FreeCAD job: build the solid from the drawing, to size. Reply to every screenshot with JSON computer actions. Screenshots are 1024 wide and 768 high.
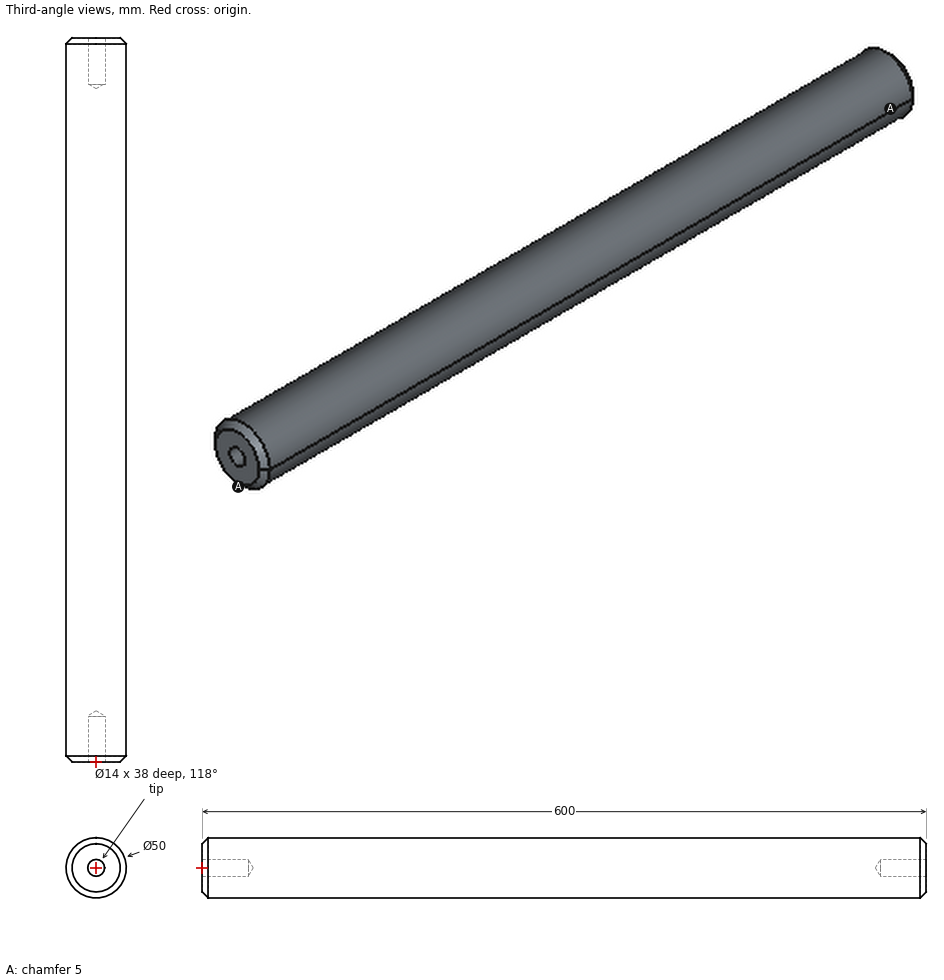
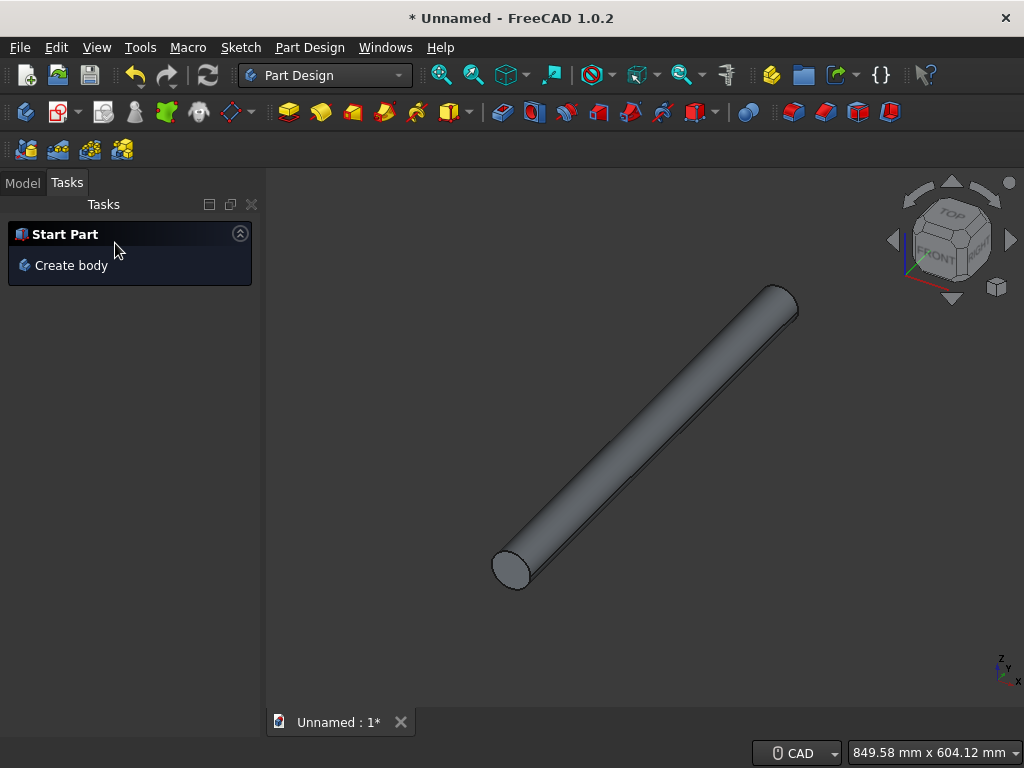
{"action": "left_click", "coordinate": [496, 554]}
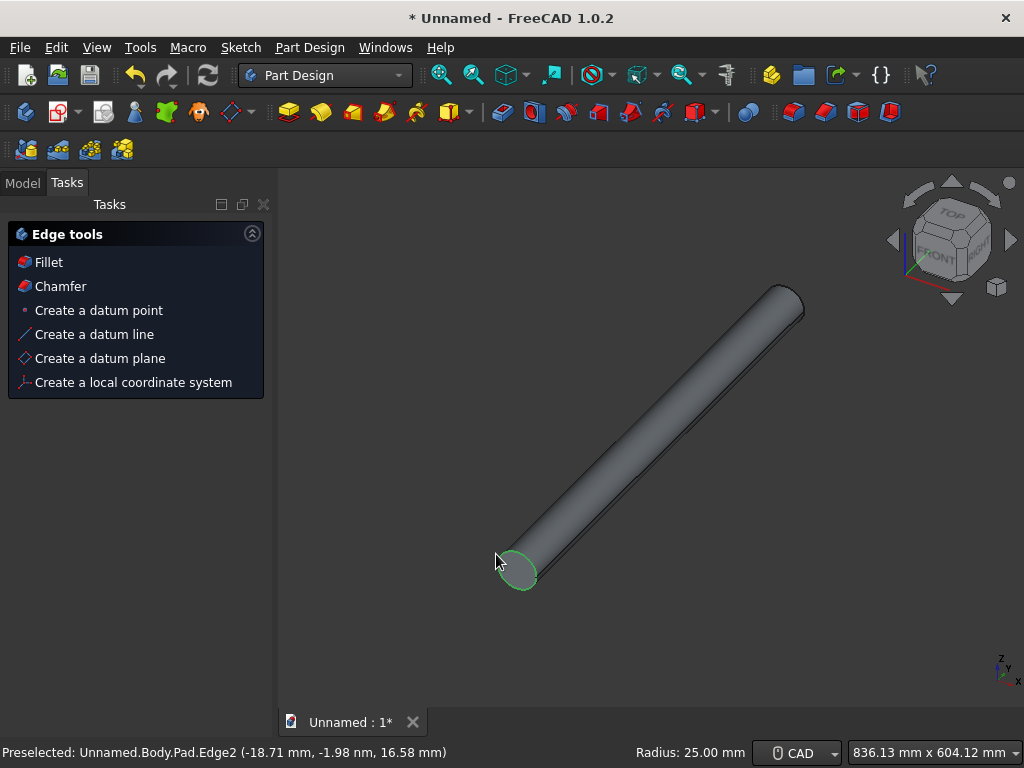
{"action": "left_click", "coordinate": [779, 284], "text": "ctrl"}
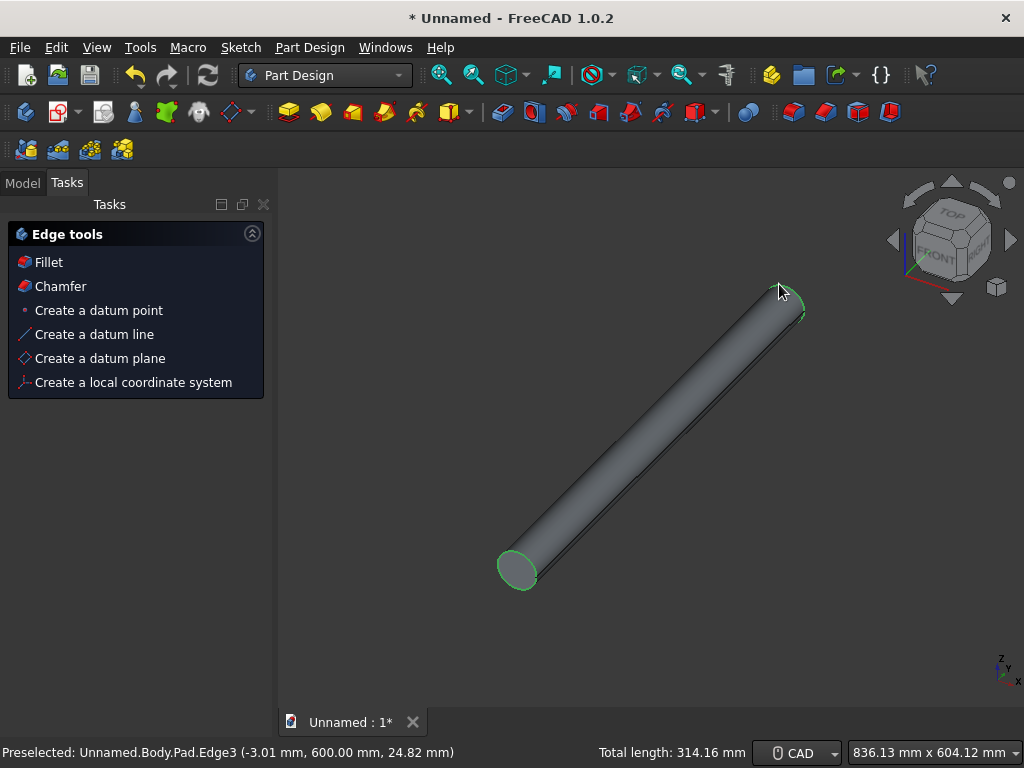
{"action": "left_click", "coordinate": [826, 112]}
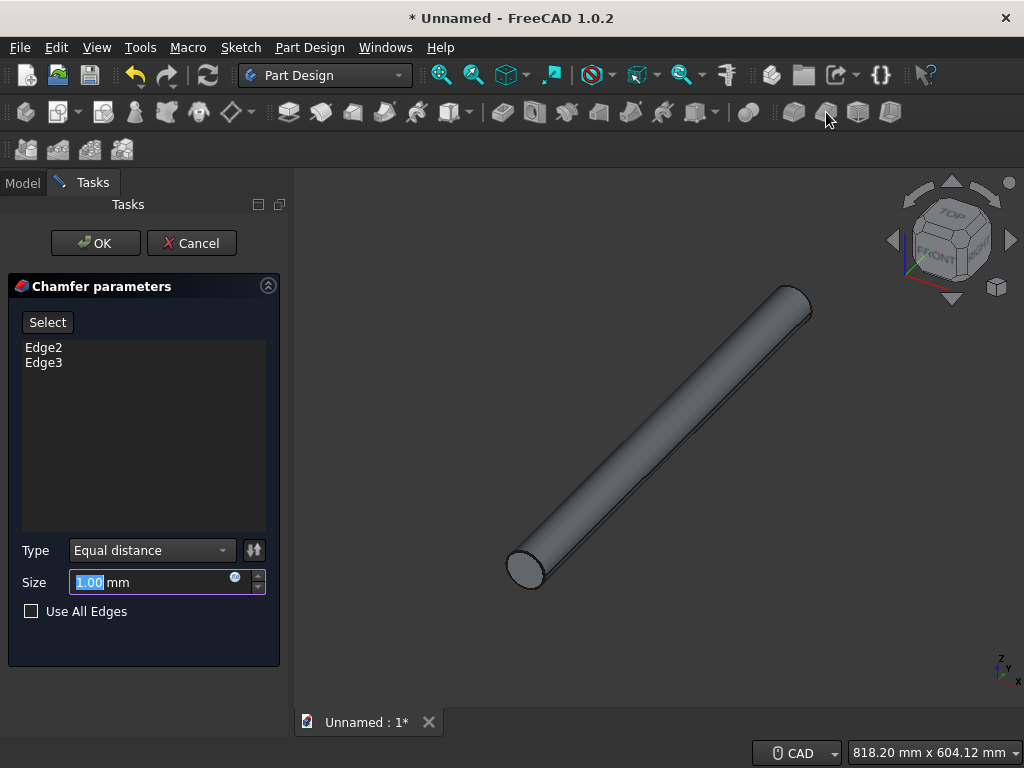
{"action": "type", "text": "5"}
{"action": "key", "text": "Tab"}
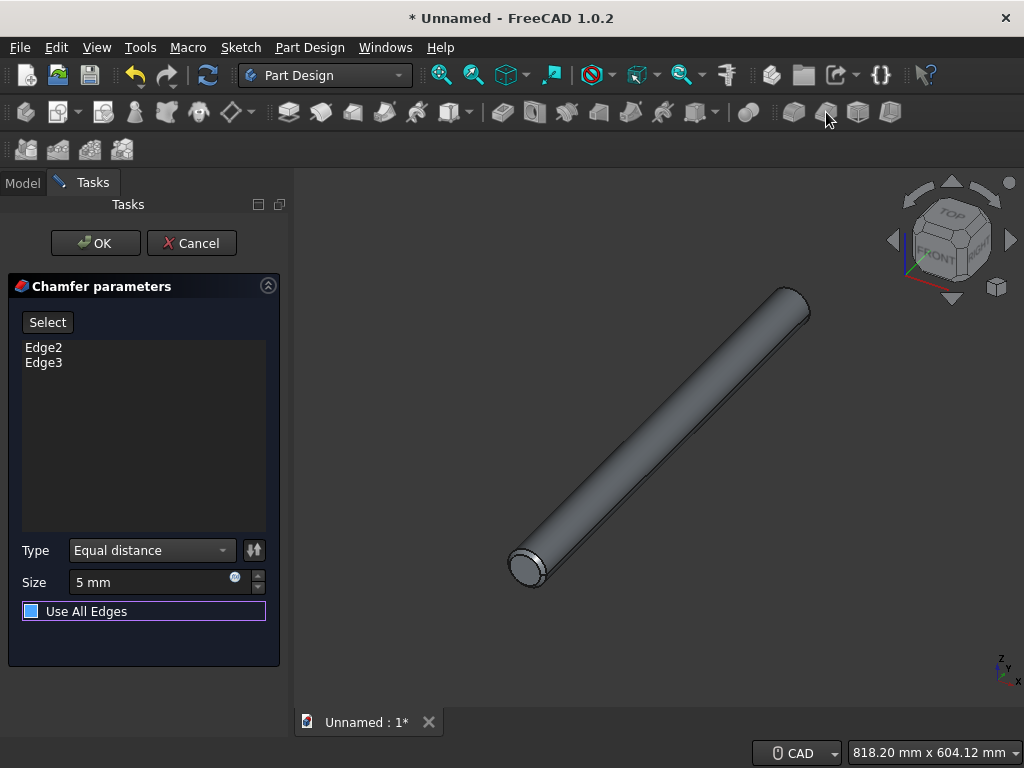
{"action": "left_click", "coordinate": [96, 243]}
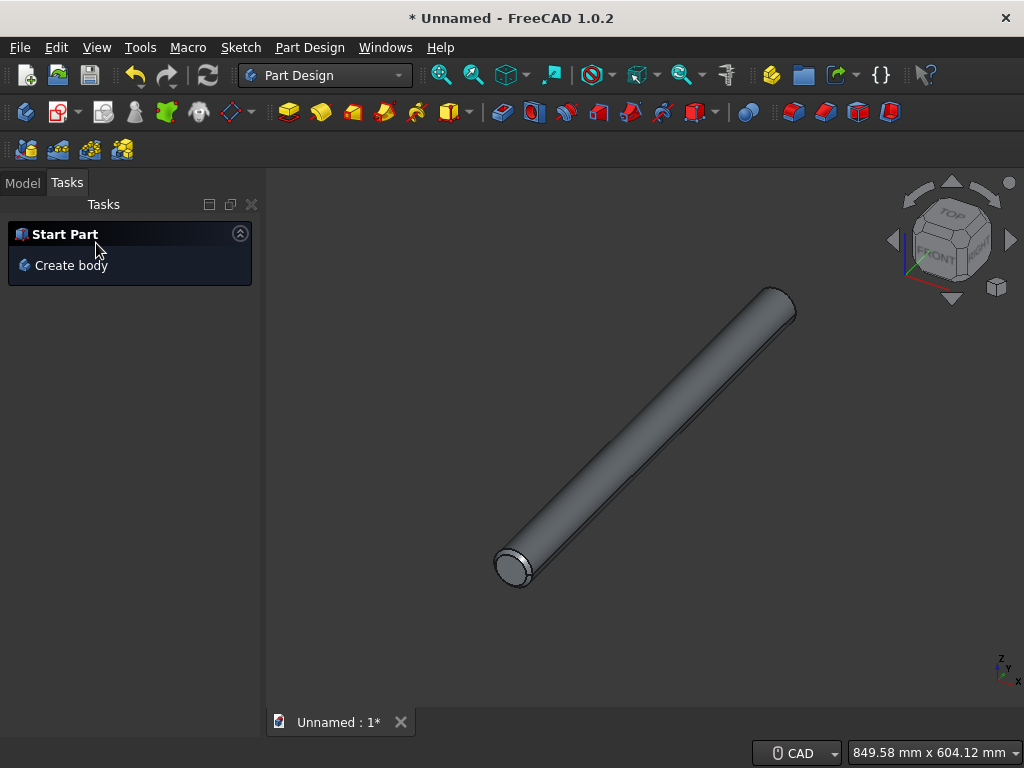
{"action": "key", "text": "4"}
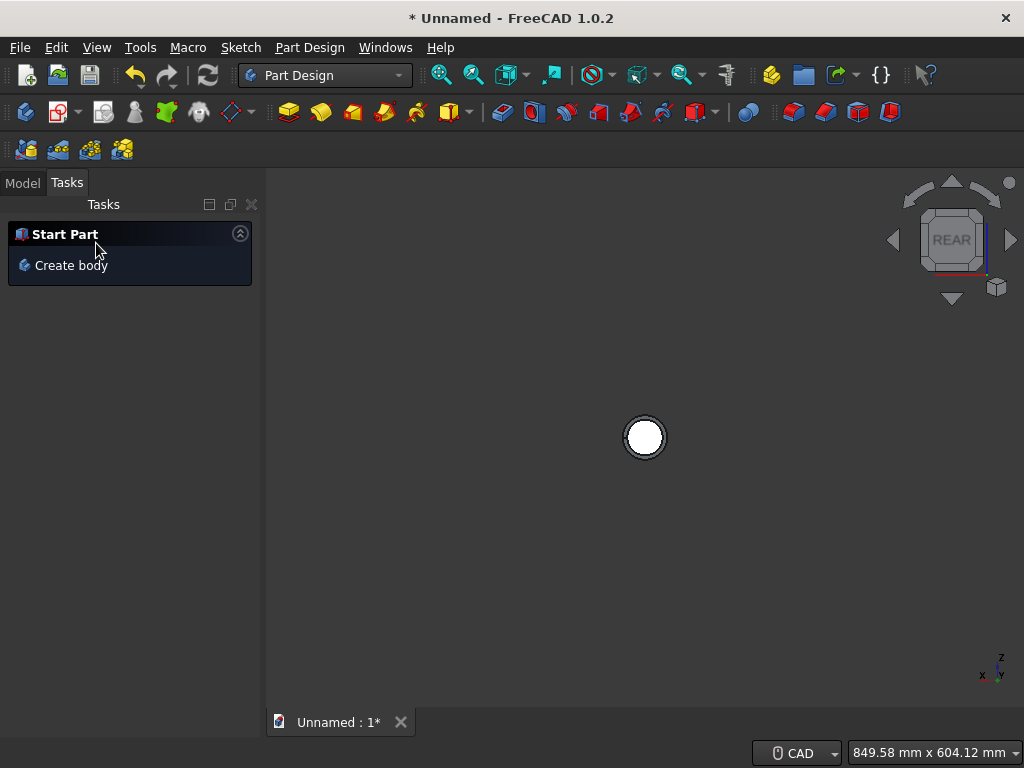
{"action": "left_click", "coordinate": [442, 76]}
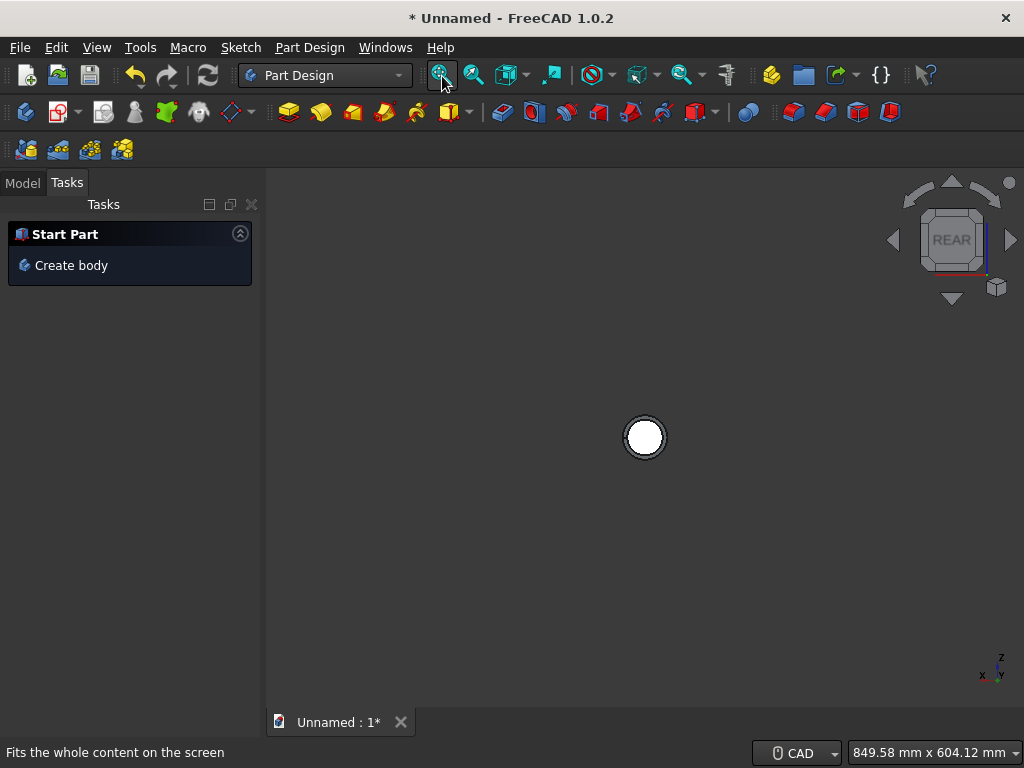
{"action": "left_click", "coordinate": [645, 437]}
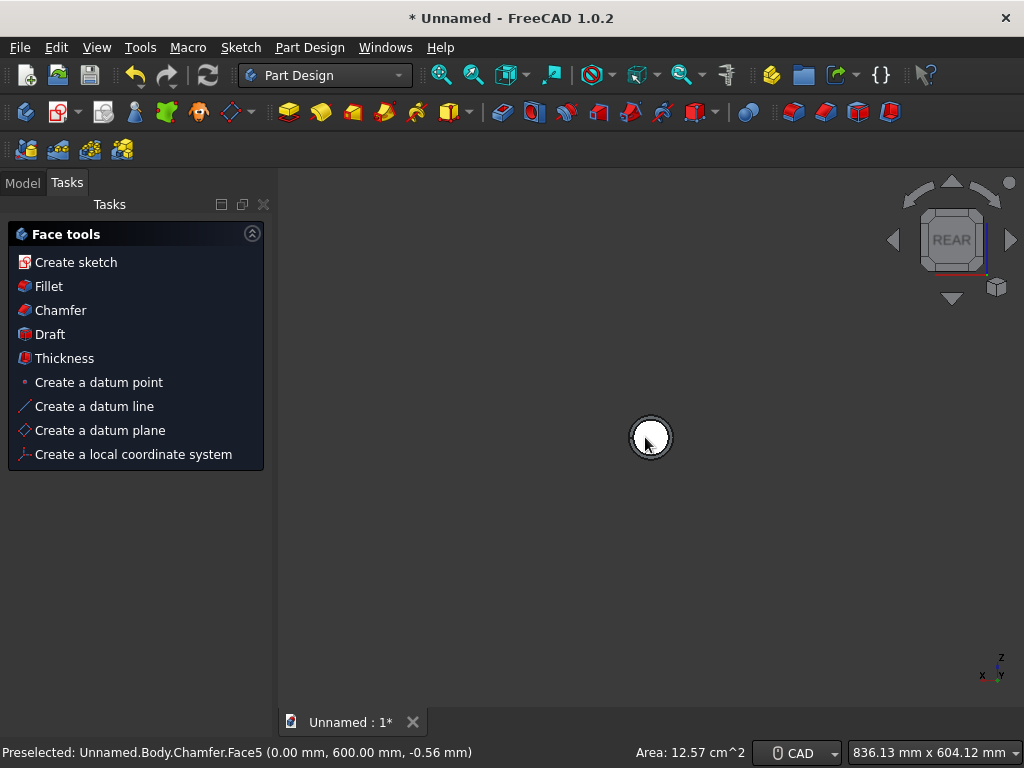
{"action": "left_click", "coordinate": [58, 112]}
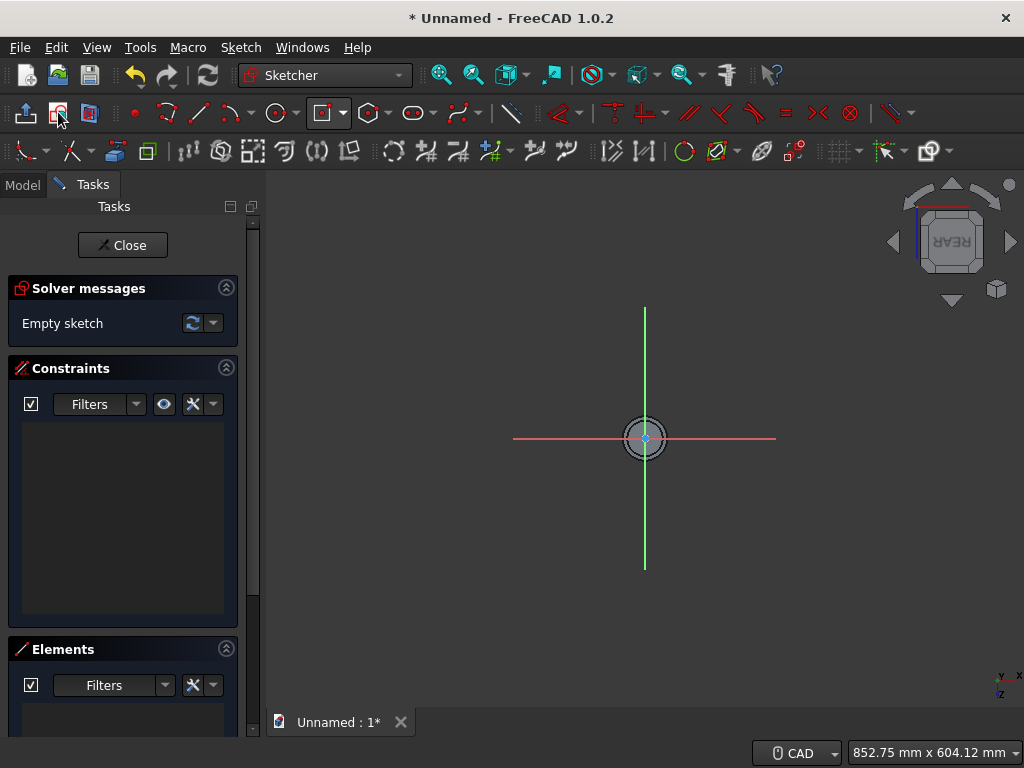
{"action": "scroll", "coordinate": [649, 438], "scroll_direction": "up", "scroll_amount": 15}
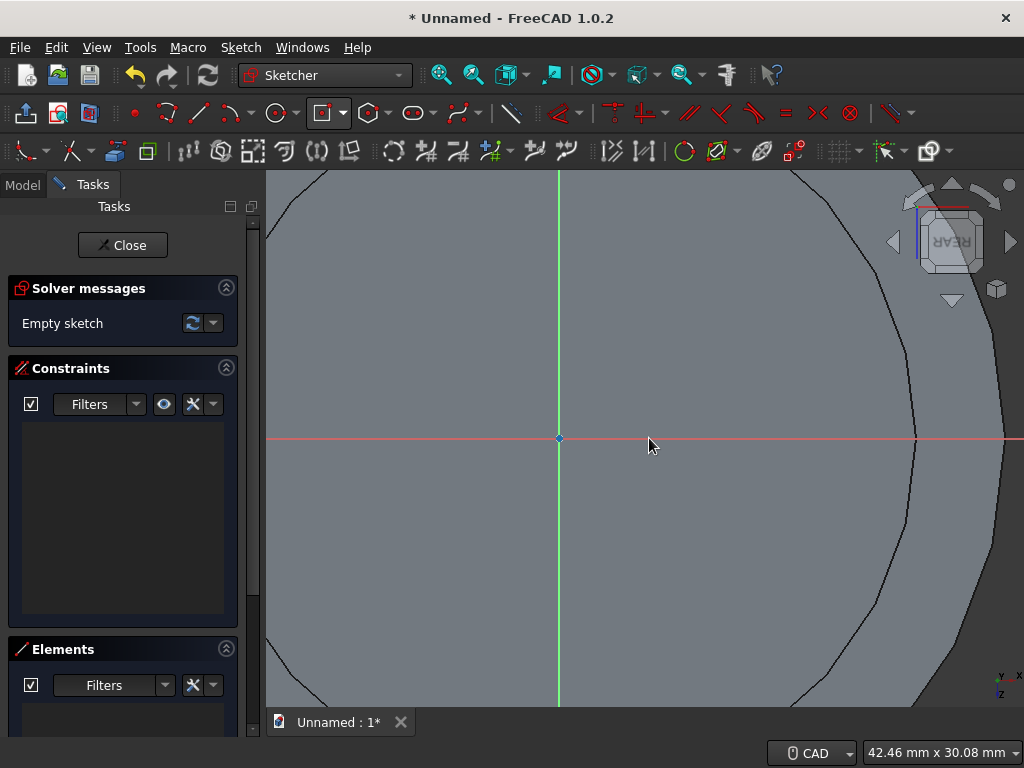
{"action": "scroll", "coordinate": [523, 438], "scroll_direction": "up", "scroll_amount": 2}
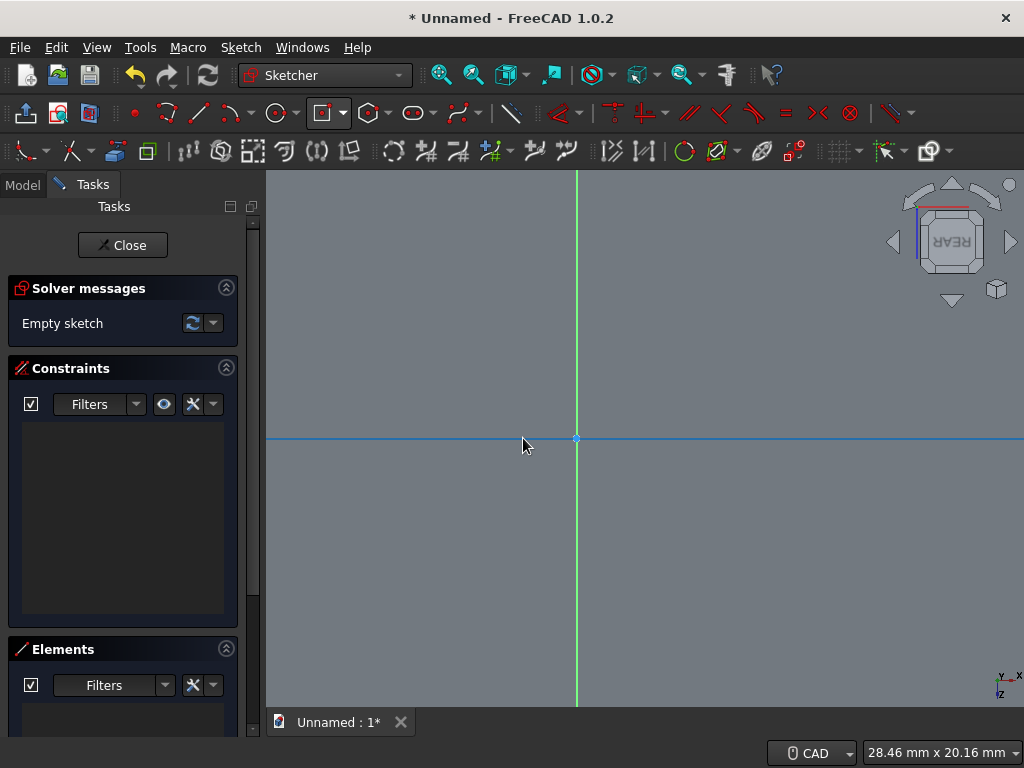
{"action": "left_click", "coordinate": [276, 114]}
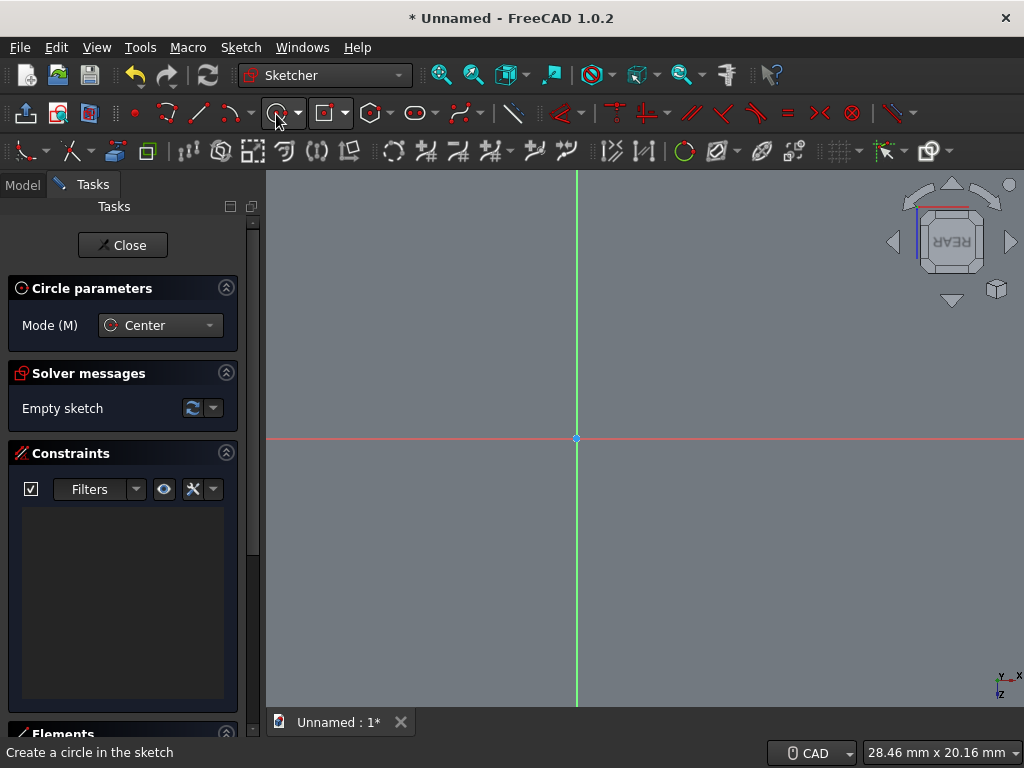
{"action": "left_click", "coordinate": [577, 438]}
{"action": "mouse_move", "coordinate": [708, 307]}